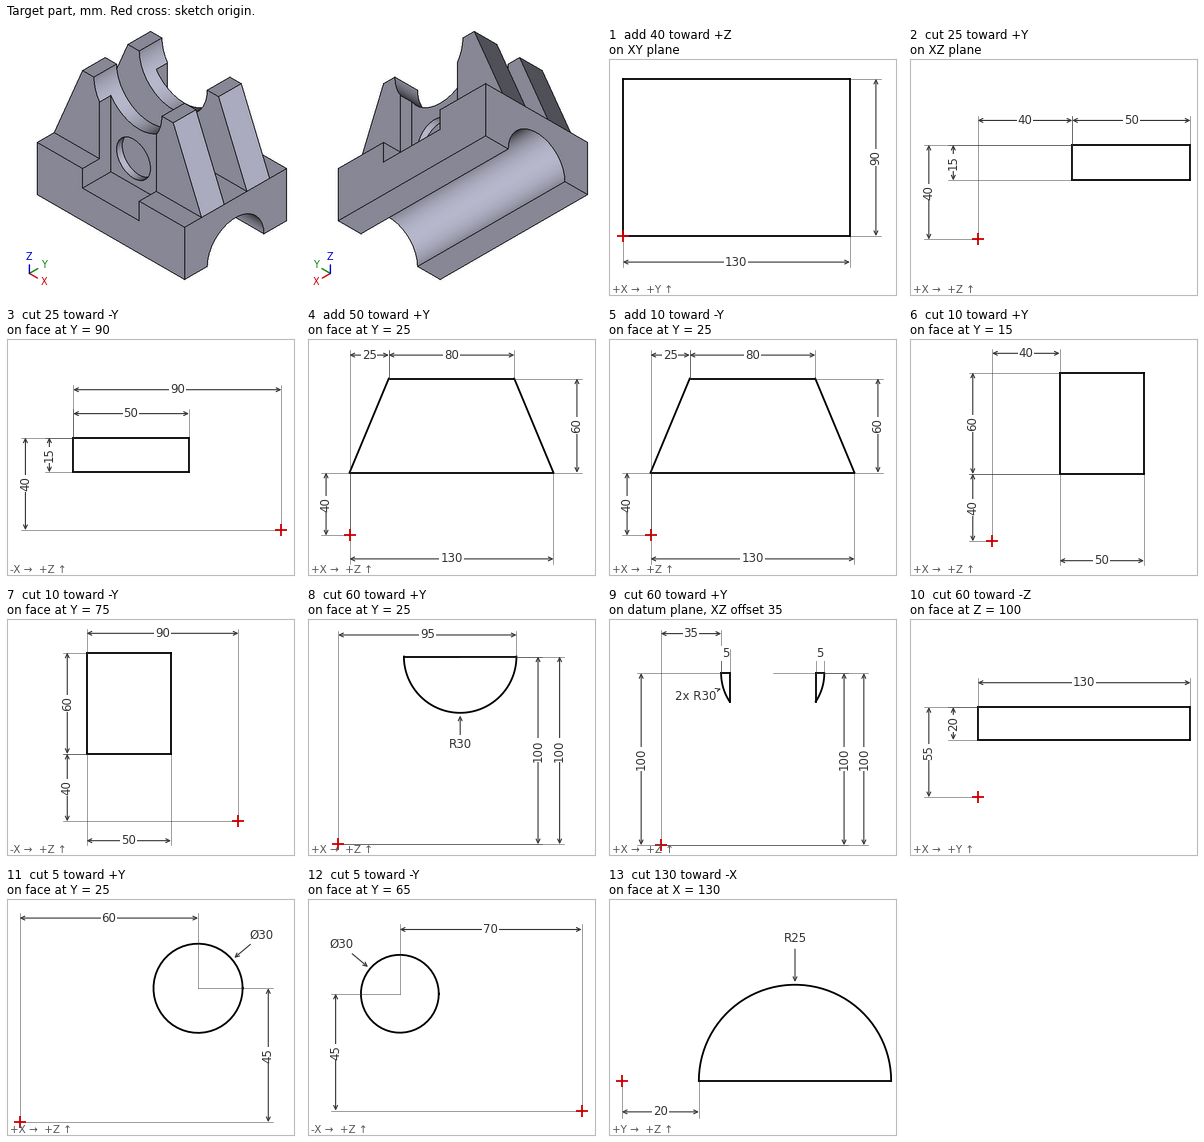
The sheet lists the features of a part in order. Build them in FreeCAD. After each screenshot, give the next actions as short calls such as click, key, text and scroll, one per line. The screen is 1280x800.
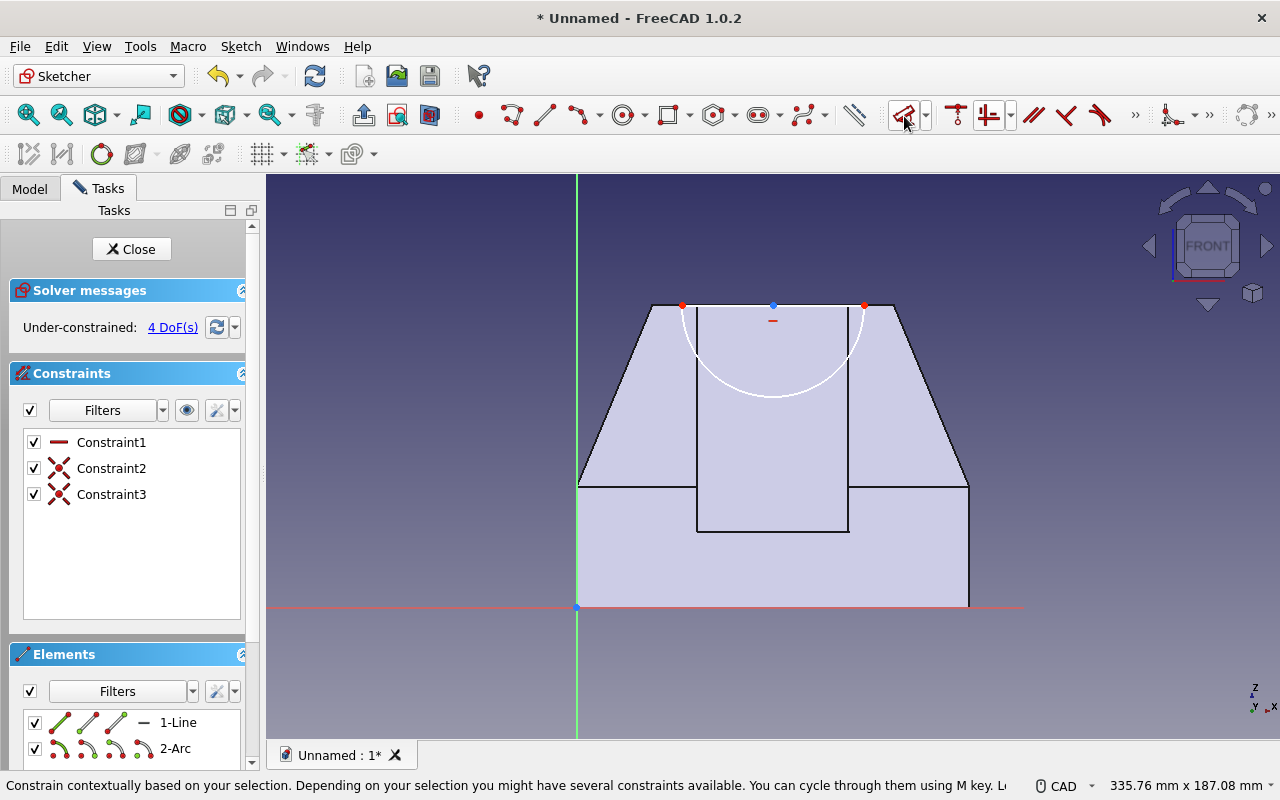
click(720, 380)
click(701, 406)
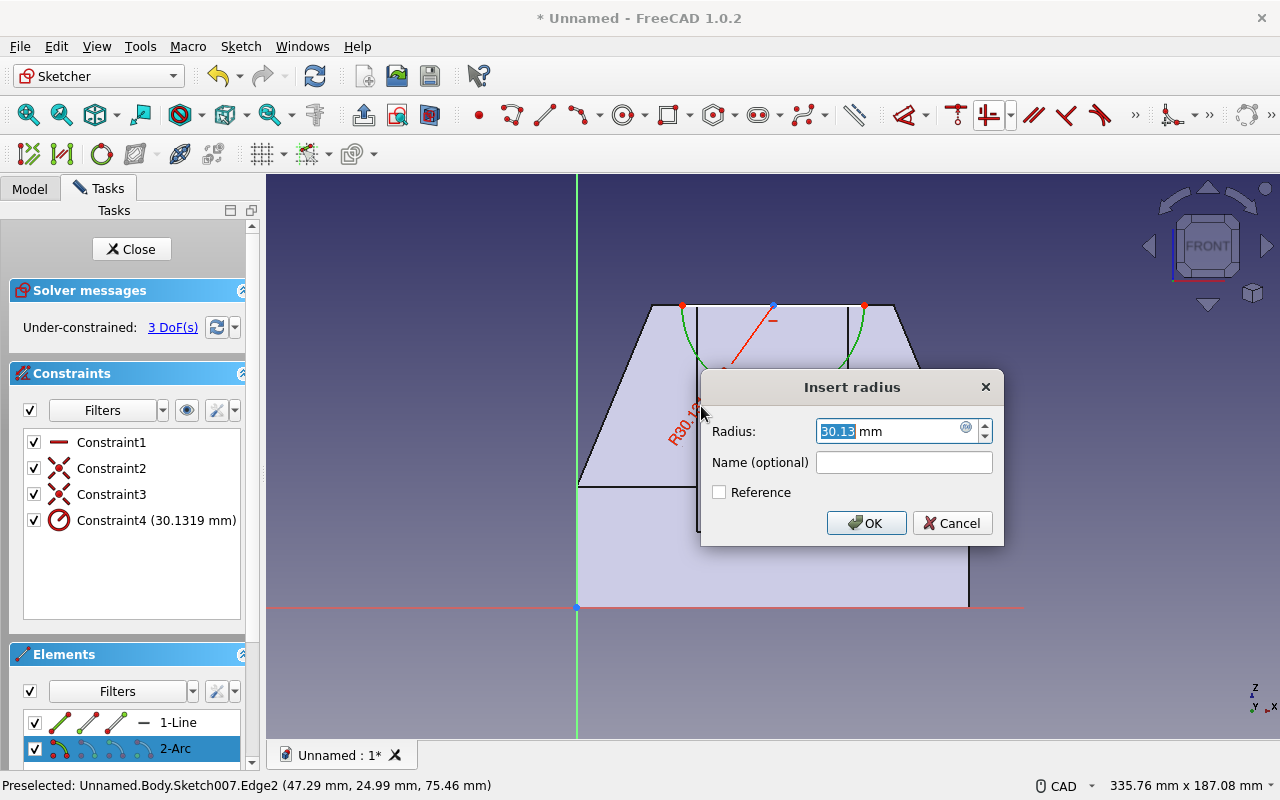
text(30)
key(Return)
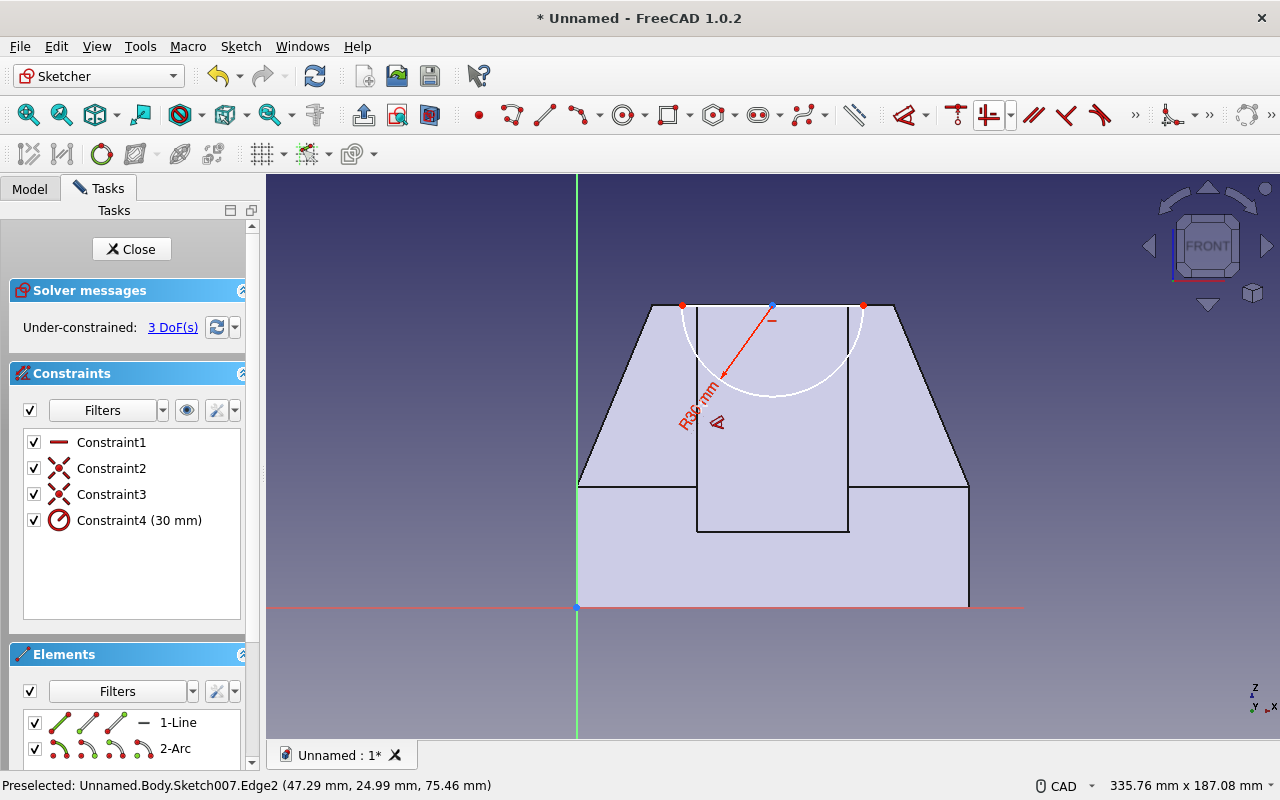
click(863, 306)
click(720, 642)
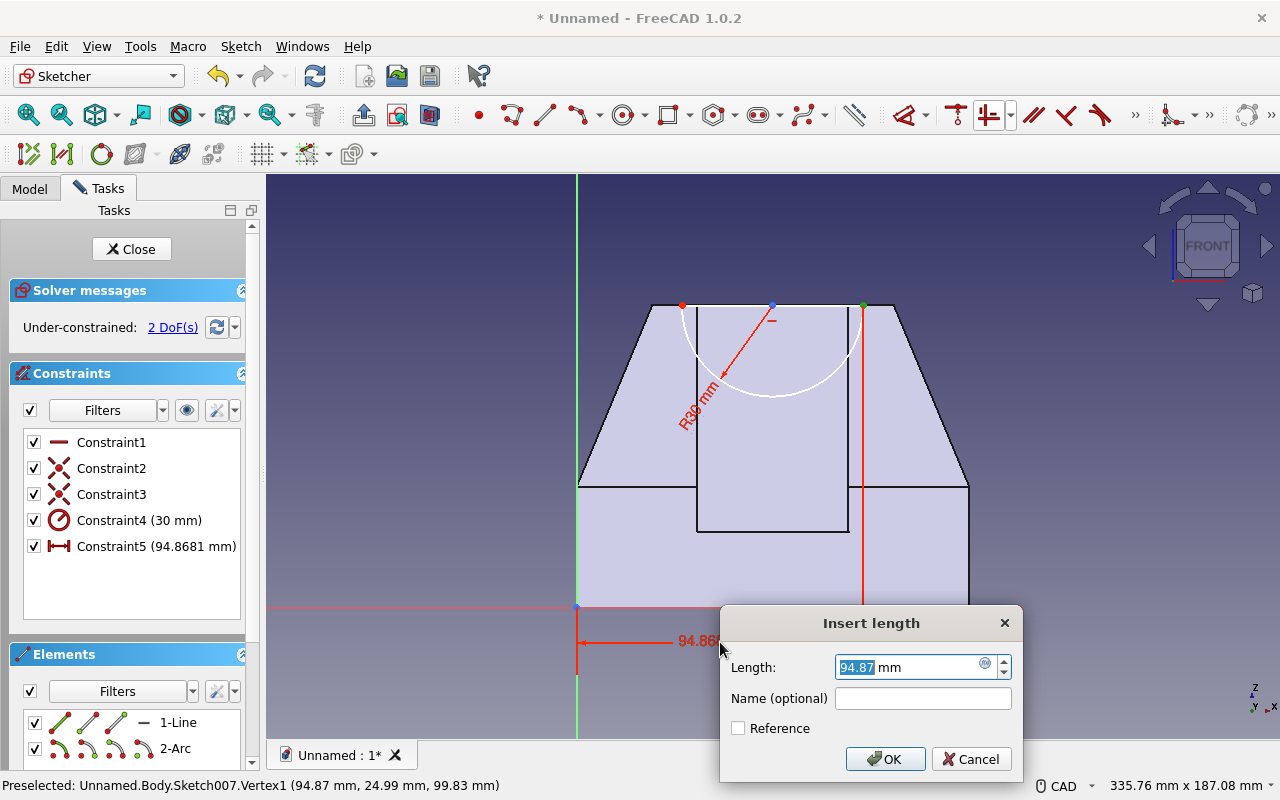
text(95)
key(Return)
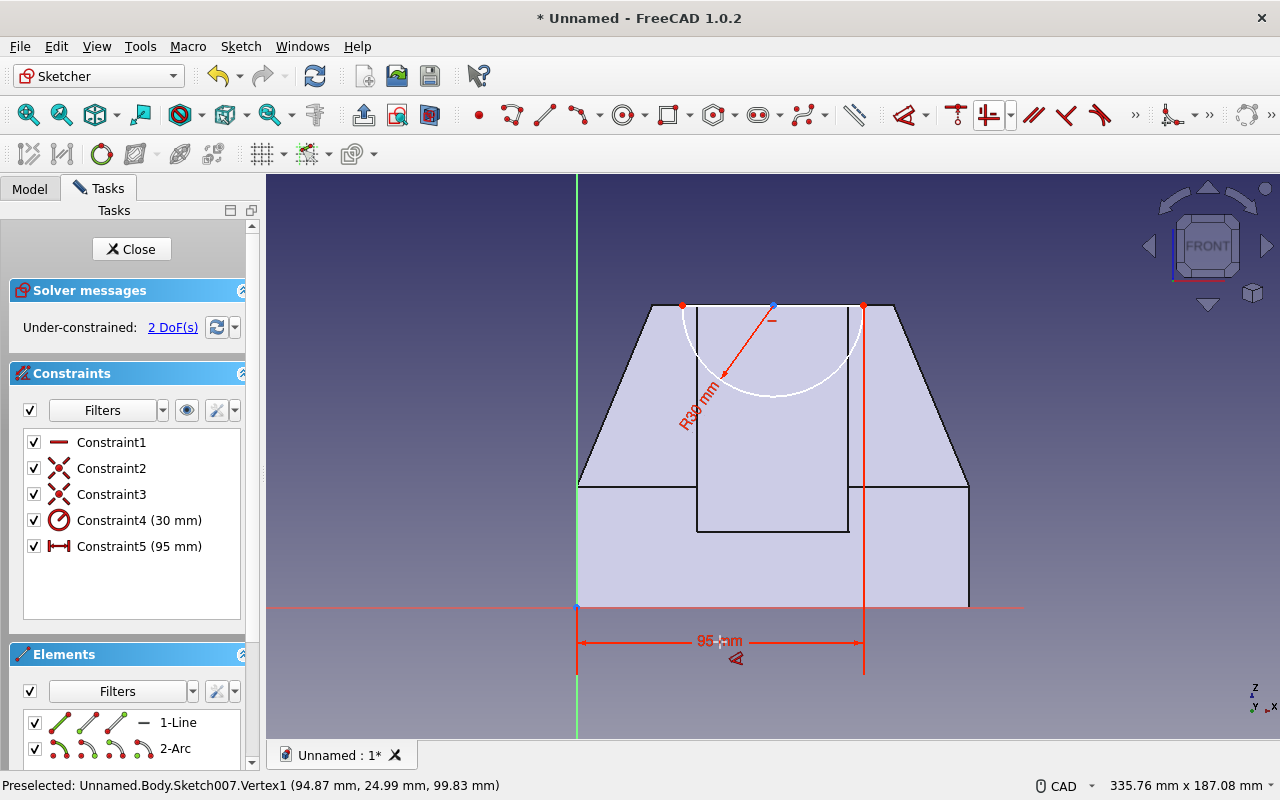
click(864, 306)
click(898, 457)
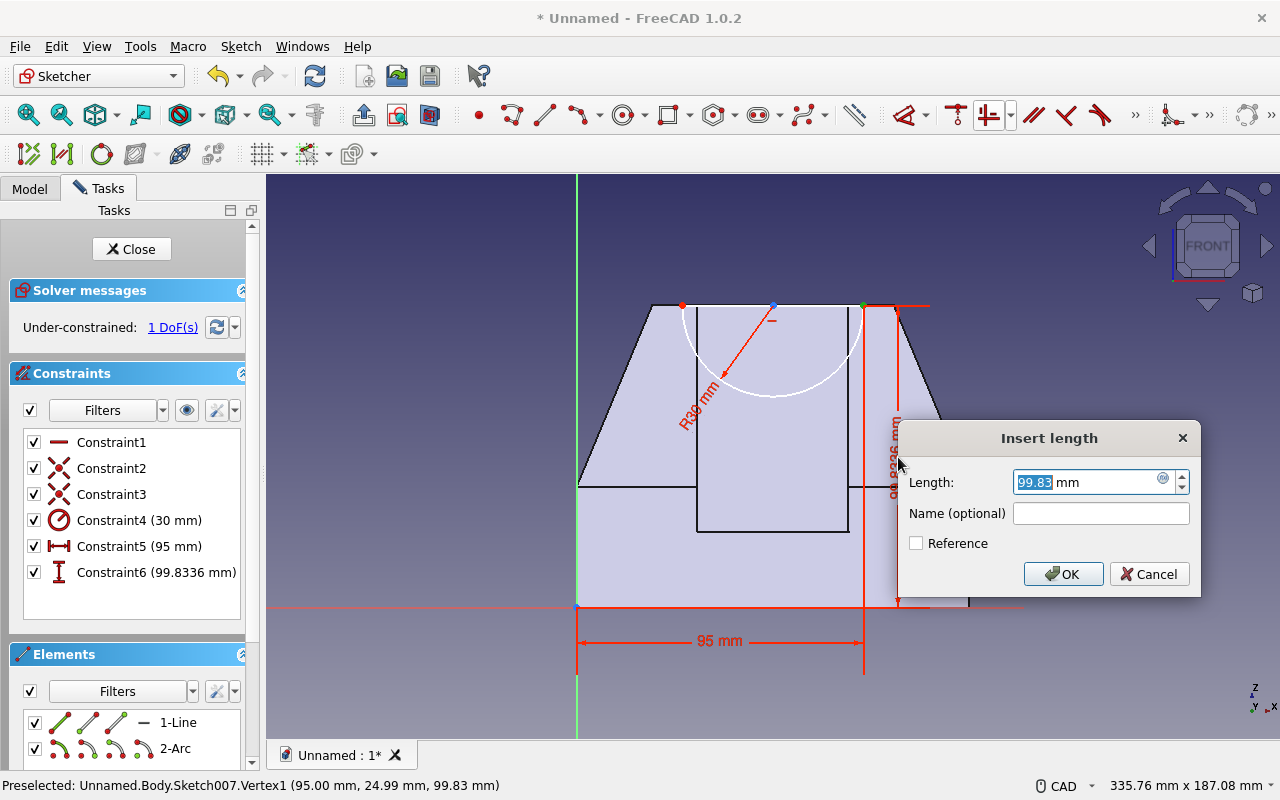
text(100)
key(Return)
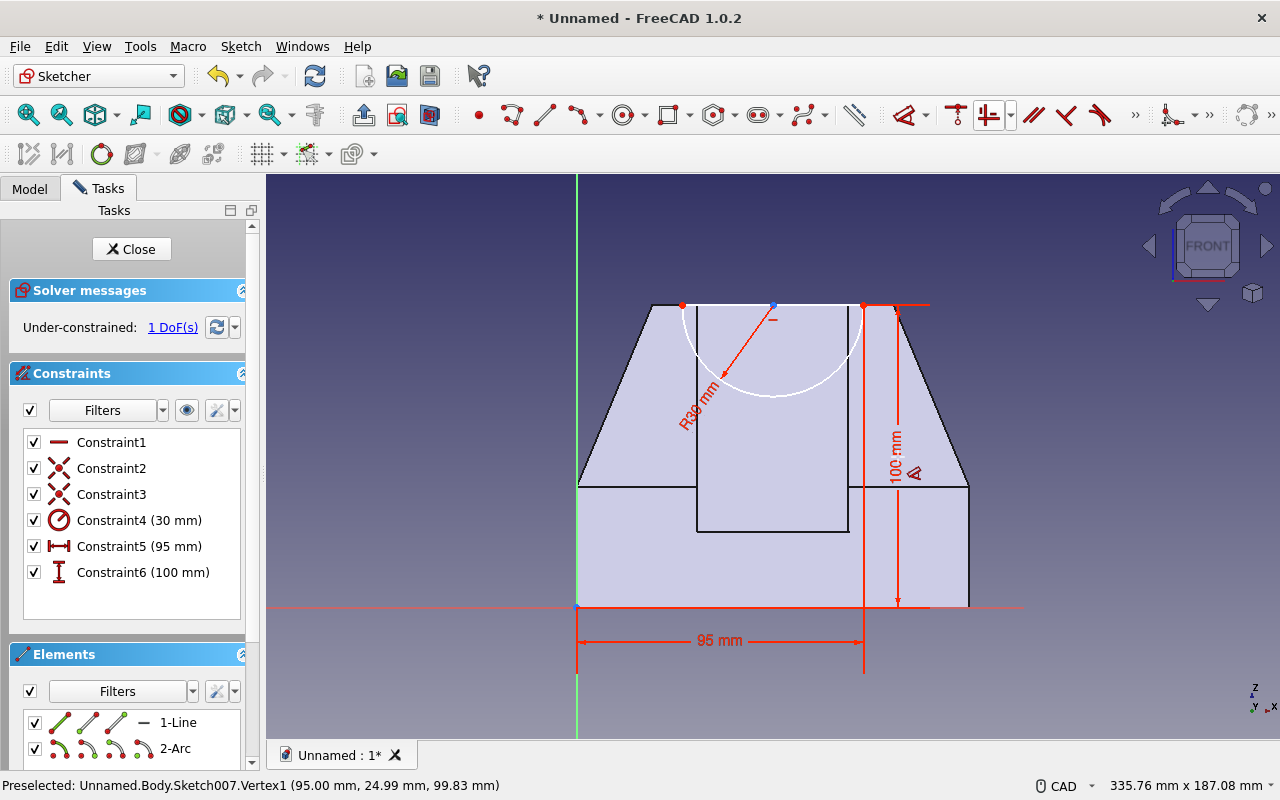
click(773, 306)
click(543, 457)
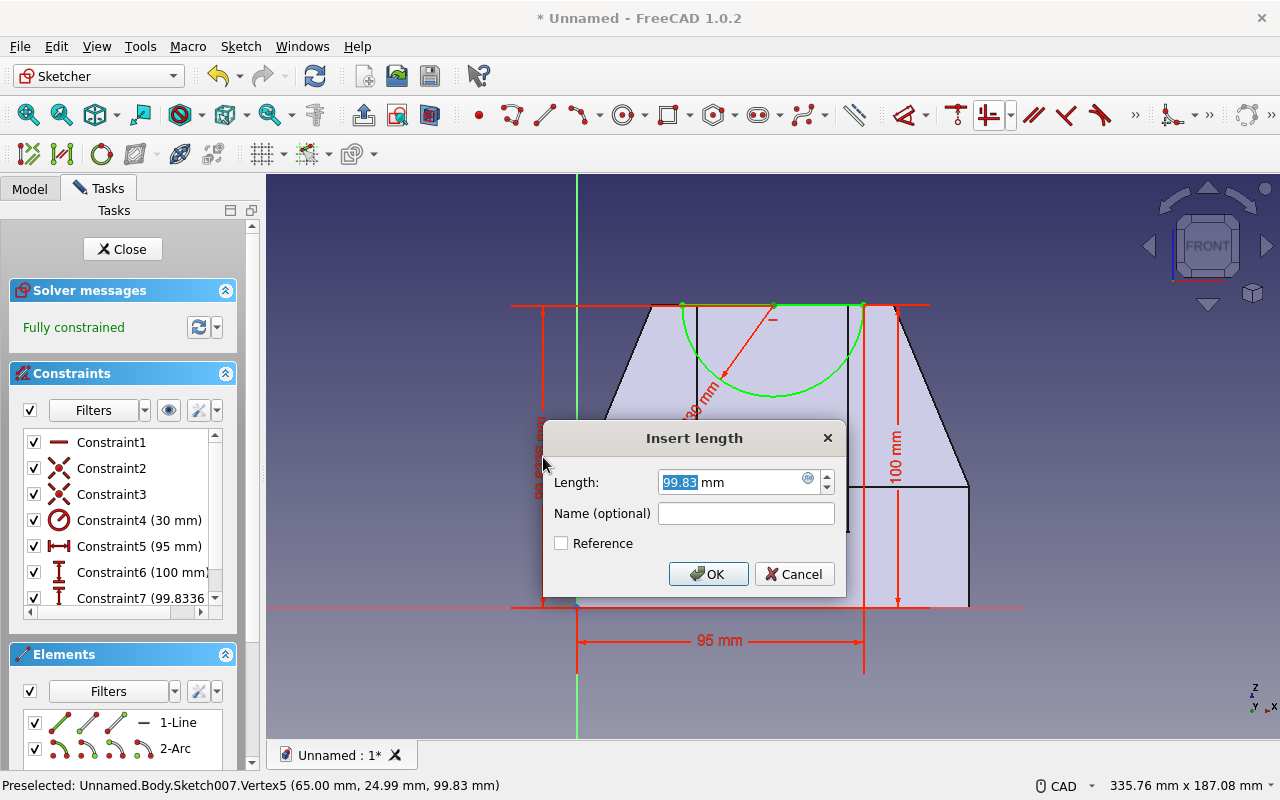
text(100)
key(Return)
key(Escape)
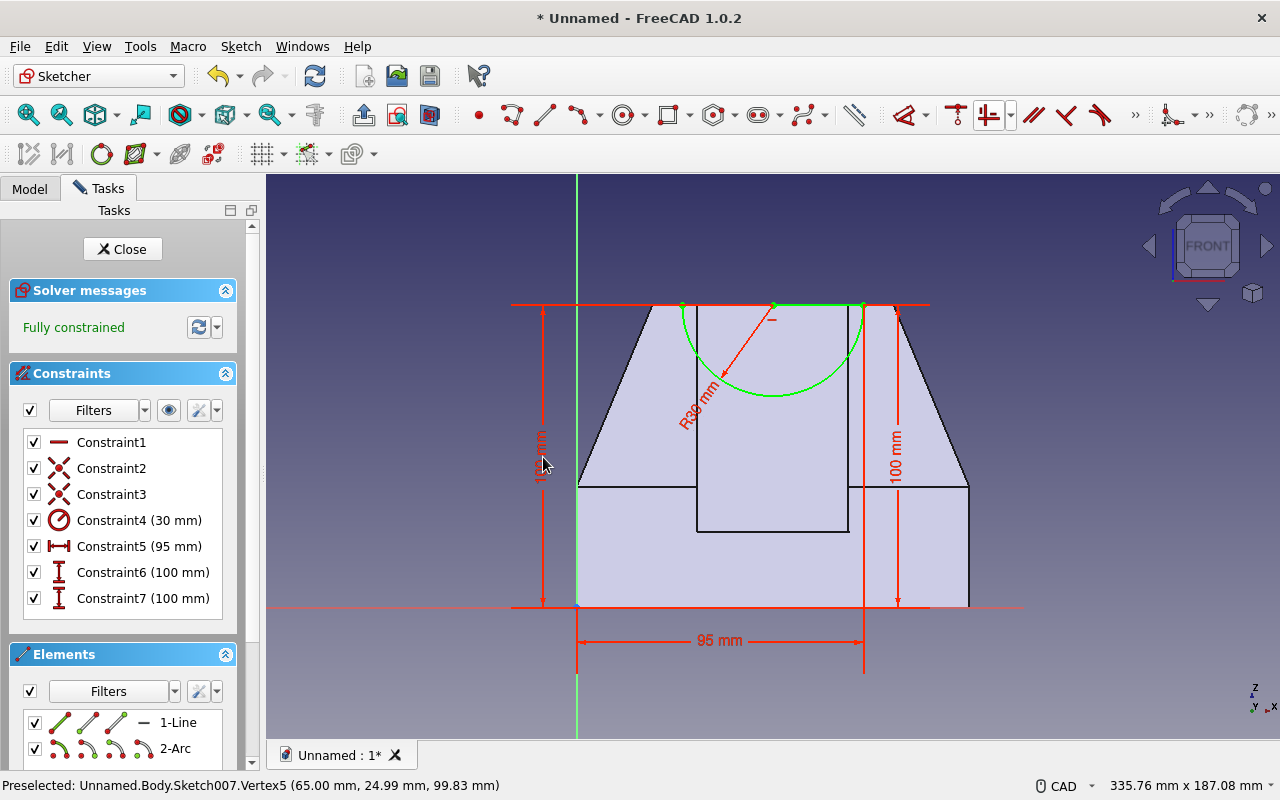
click(123, 249)